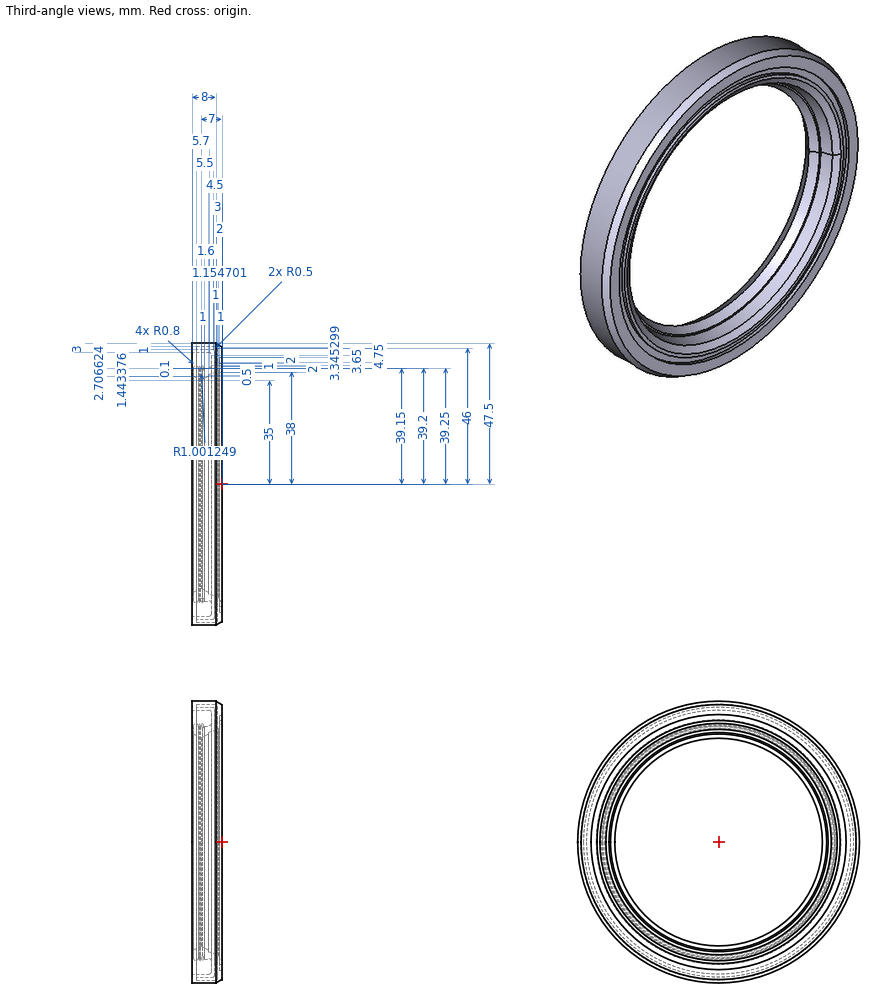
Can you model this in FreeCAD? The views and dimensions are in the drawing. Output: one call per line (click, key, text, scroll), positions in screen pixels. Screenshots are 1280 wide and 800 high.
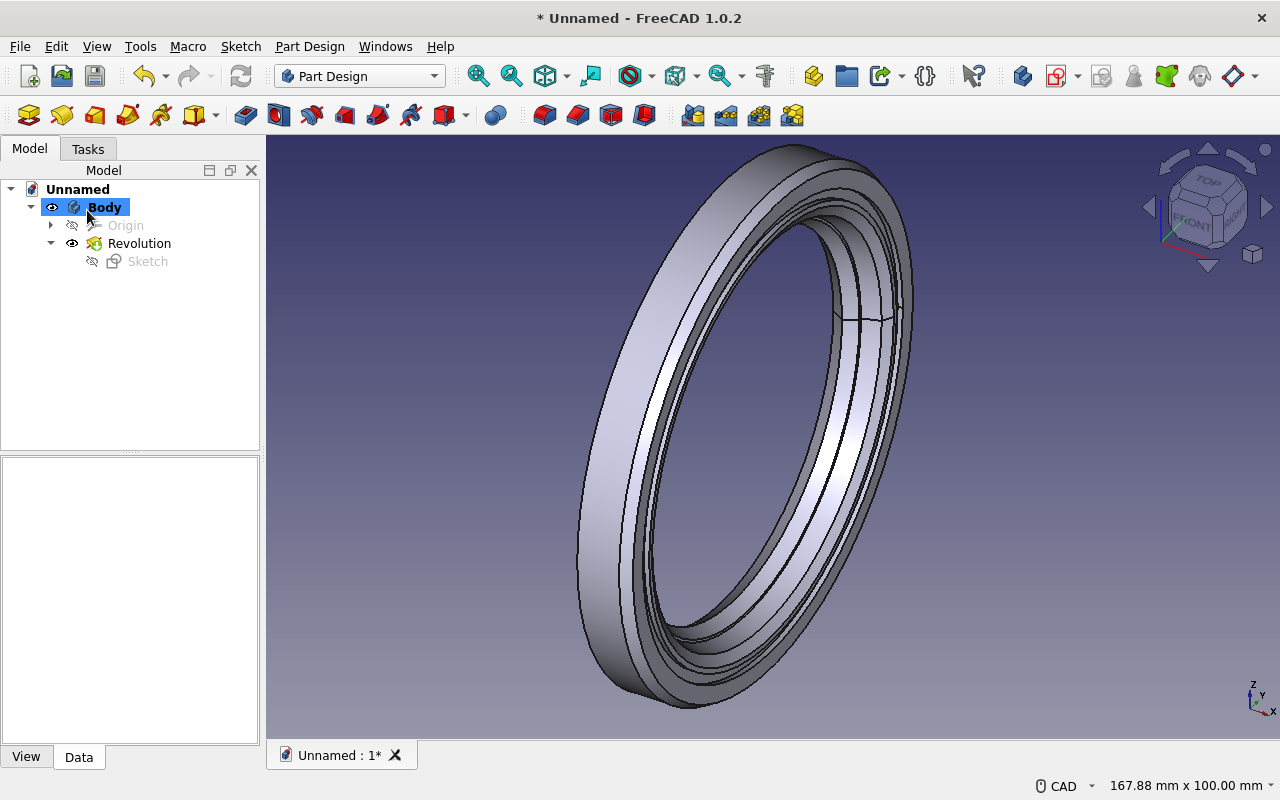
key(0)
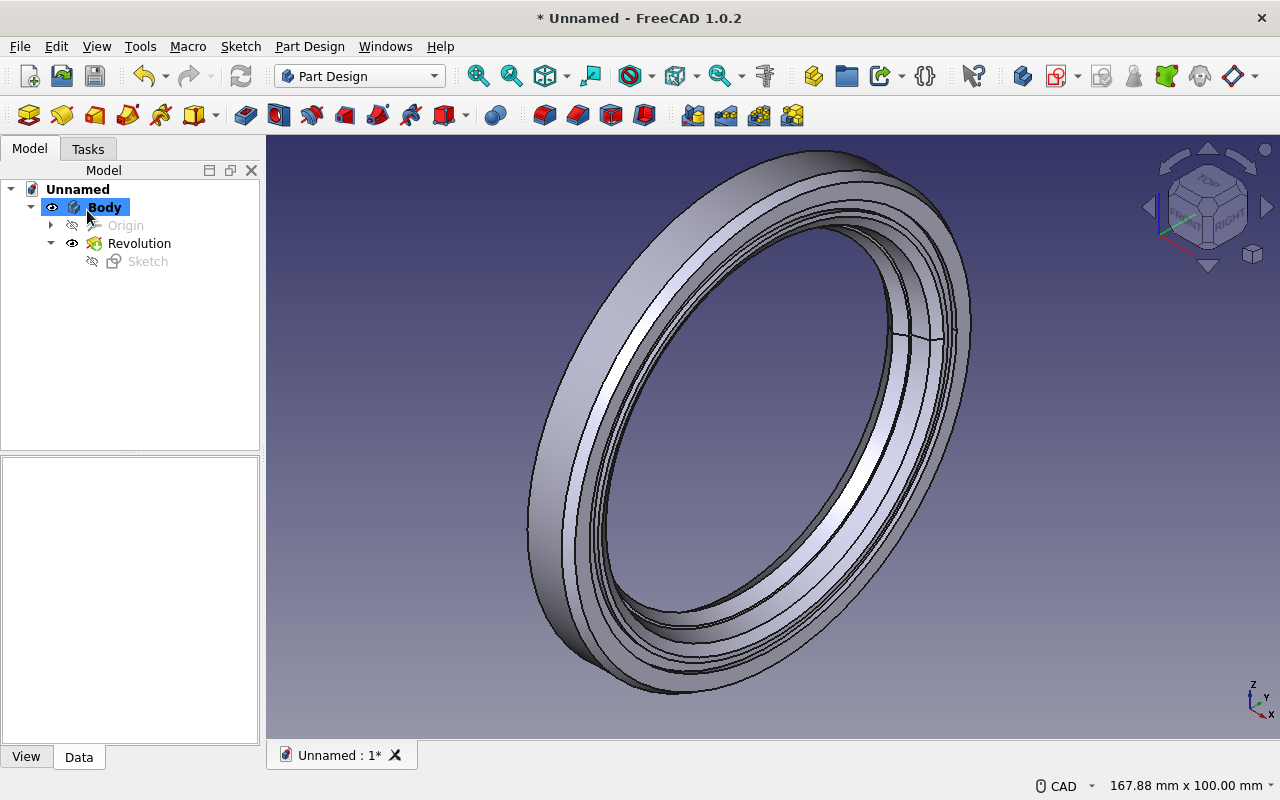
key(v)
key(f)